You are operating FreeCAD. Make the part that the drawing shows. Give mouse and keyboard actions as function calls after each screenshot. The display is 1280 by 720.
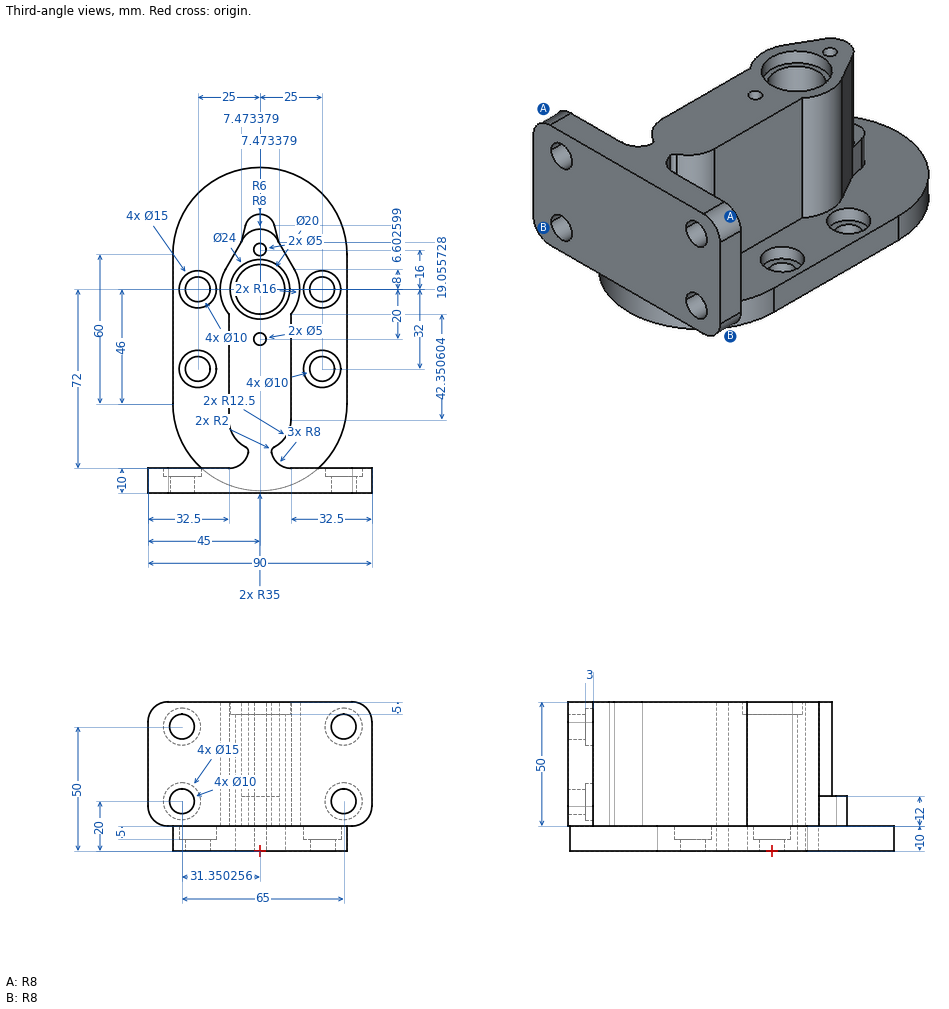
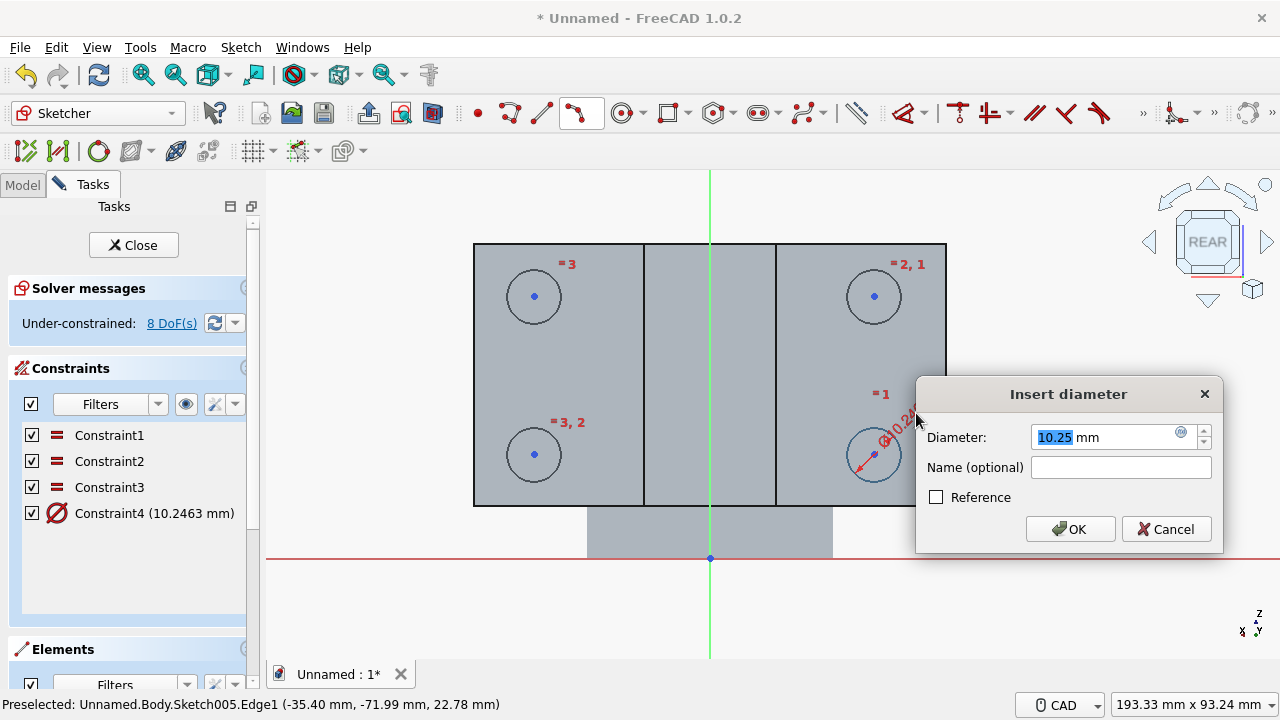
text(10)
key(Return)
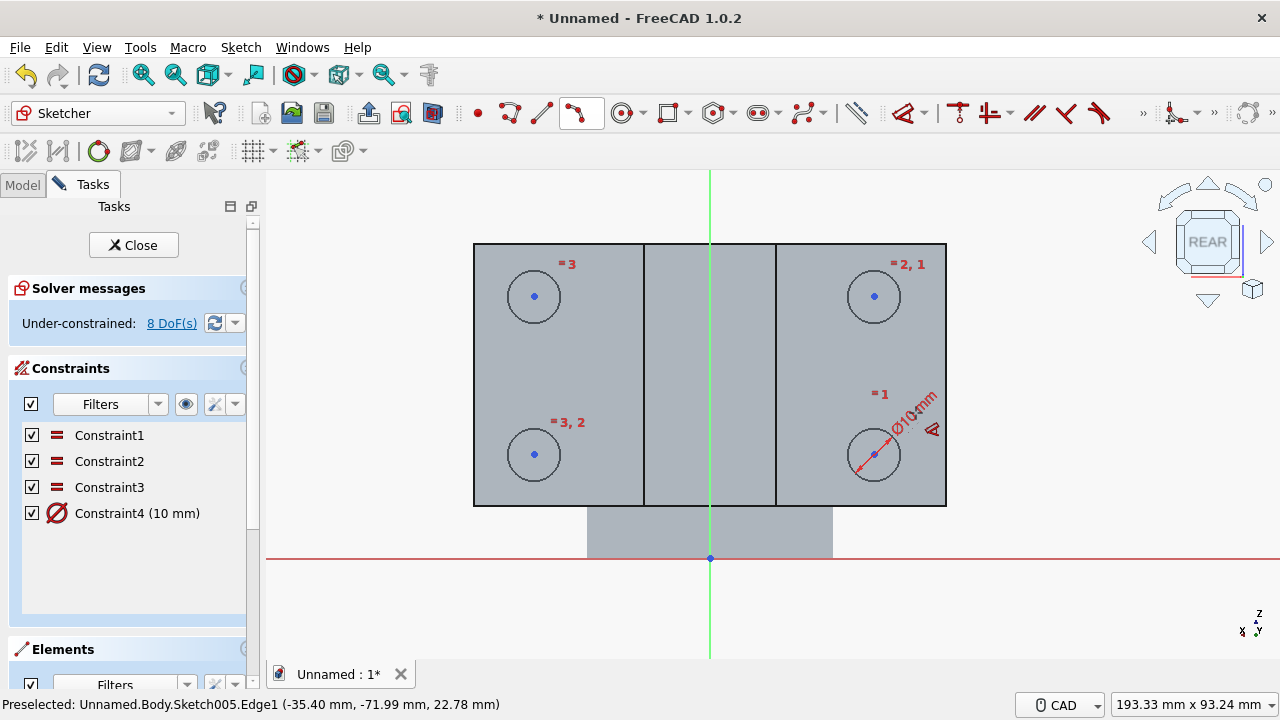
click(874, 455)
click(908, 507)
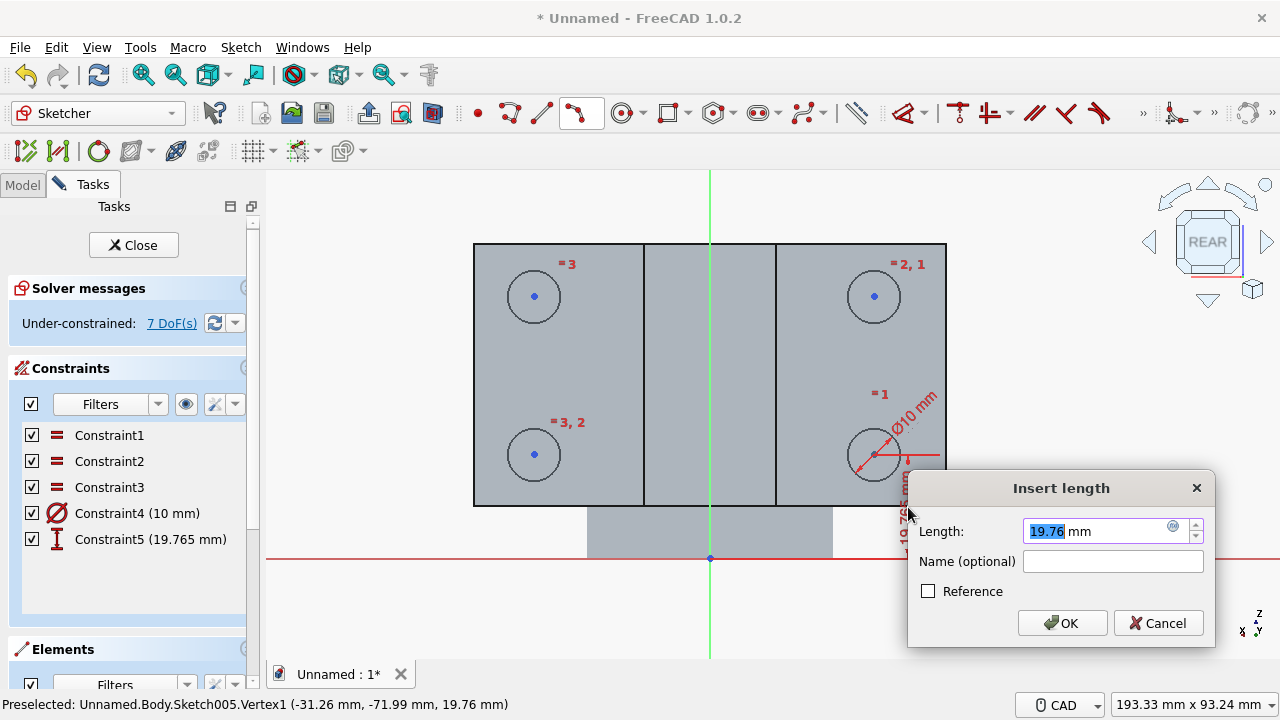
text(20)
key(Return)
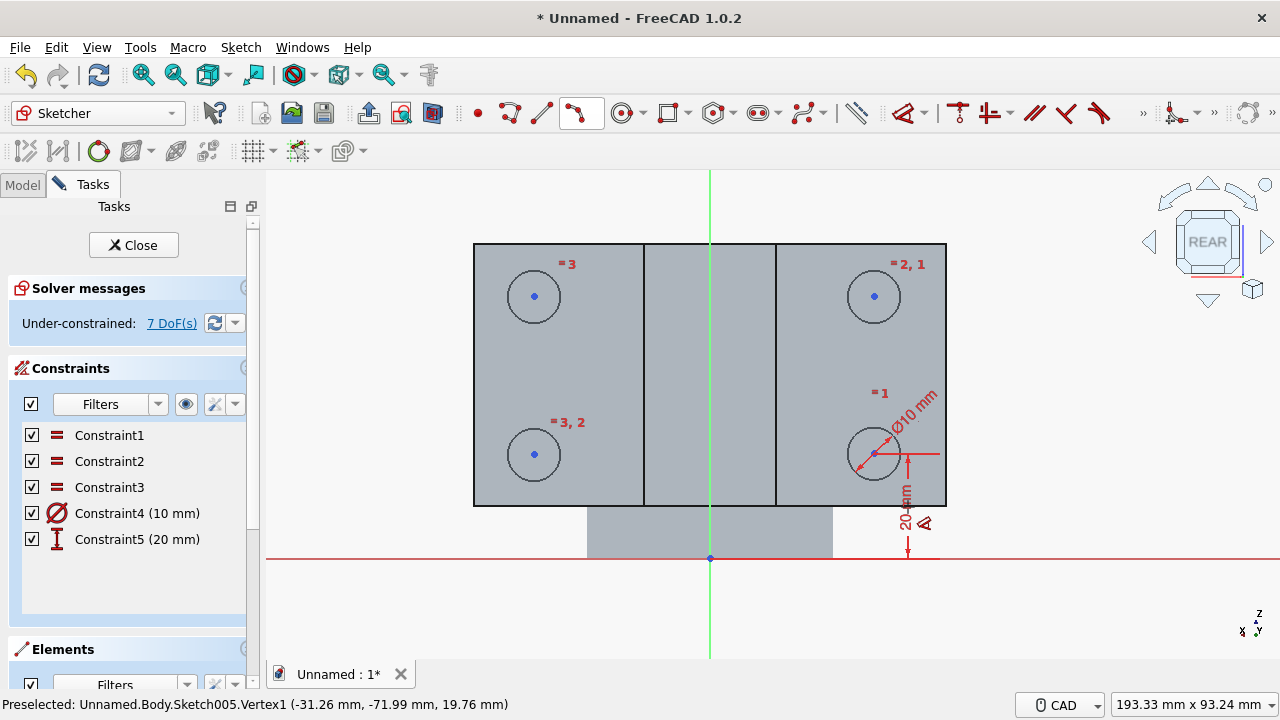
click(874, 297)
click(908, 368)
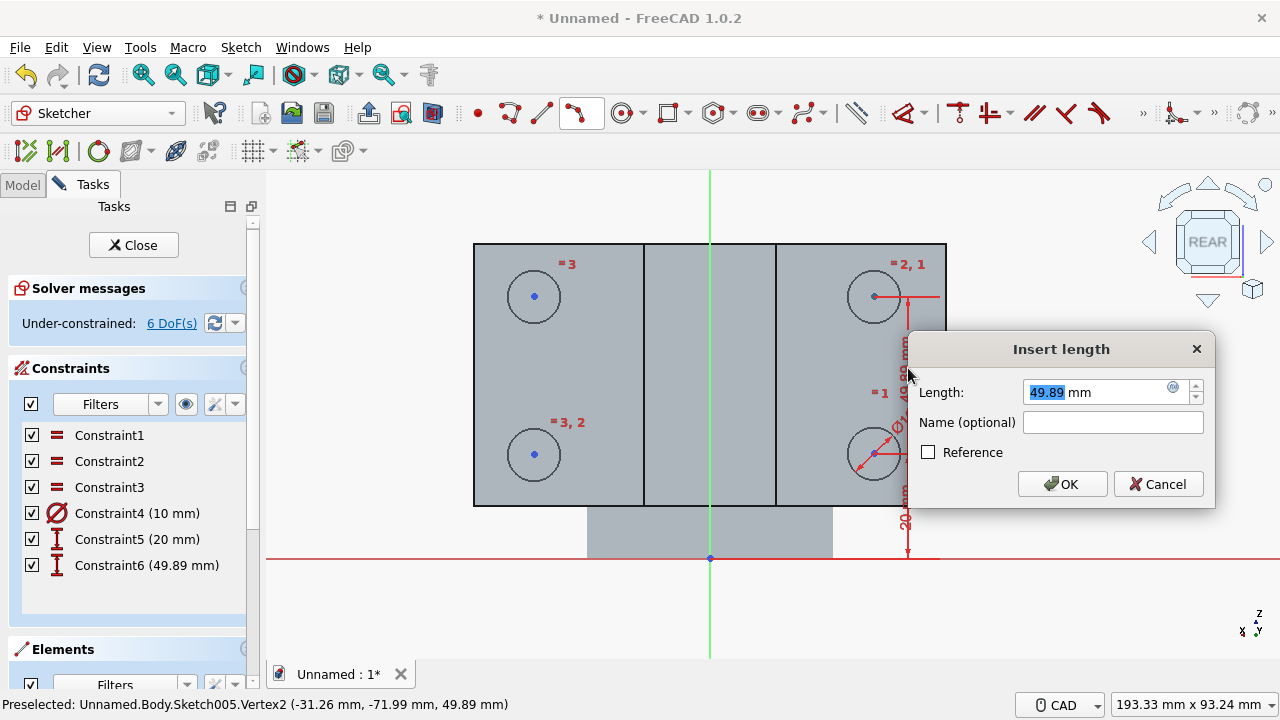
text(50)
key(Return)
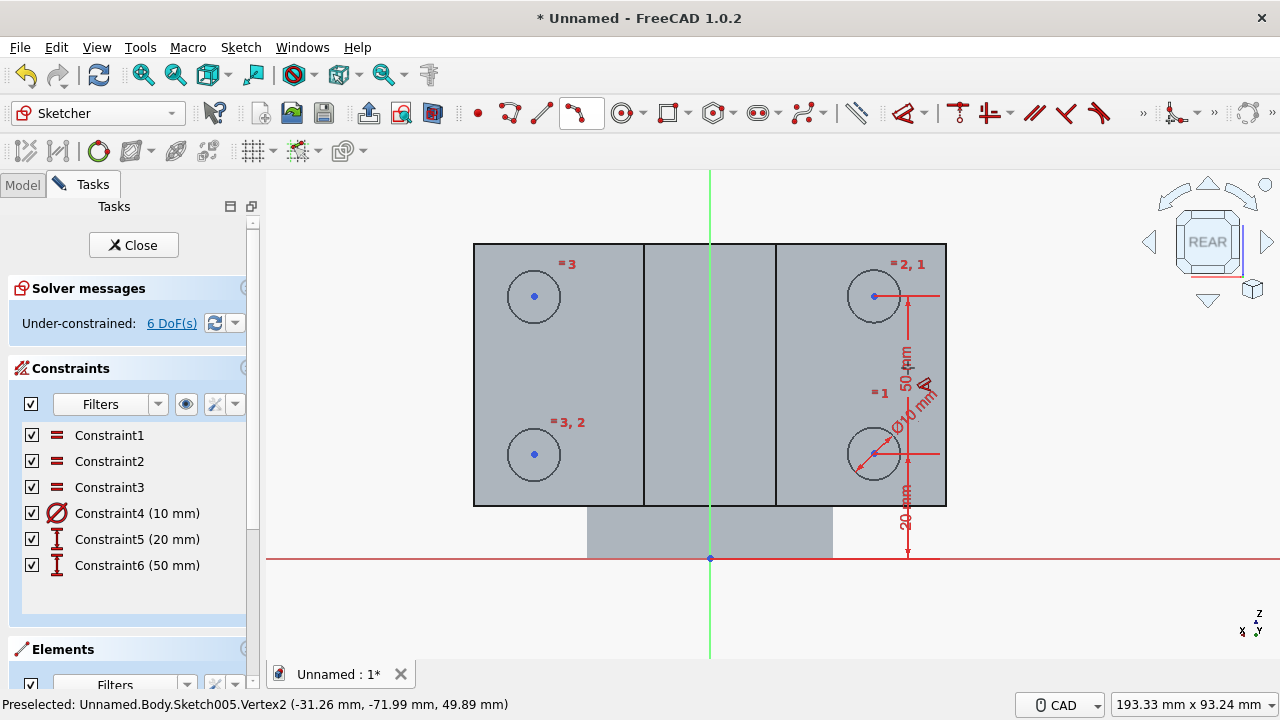
click(534, 455)
click(500, 507)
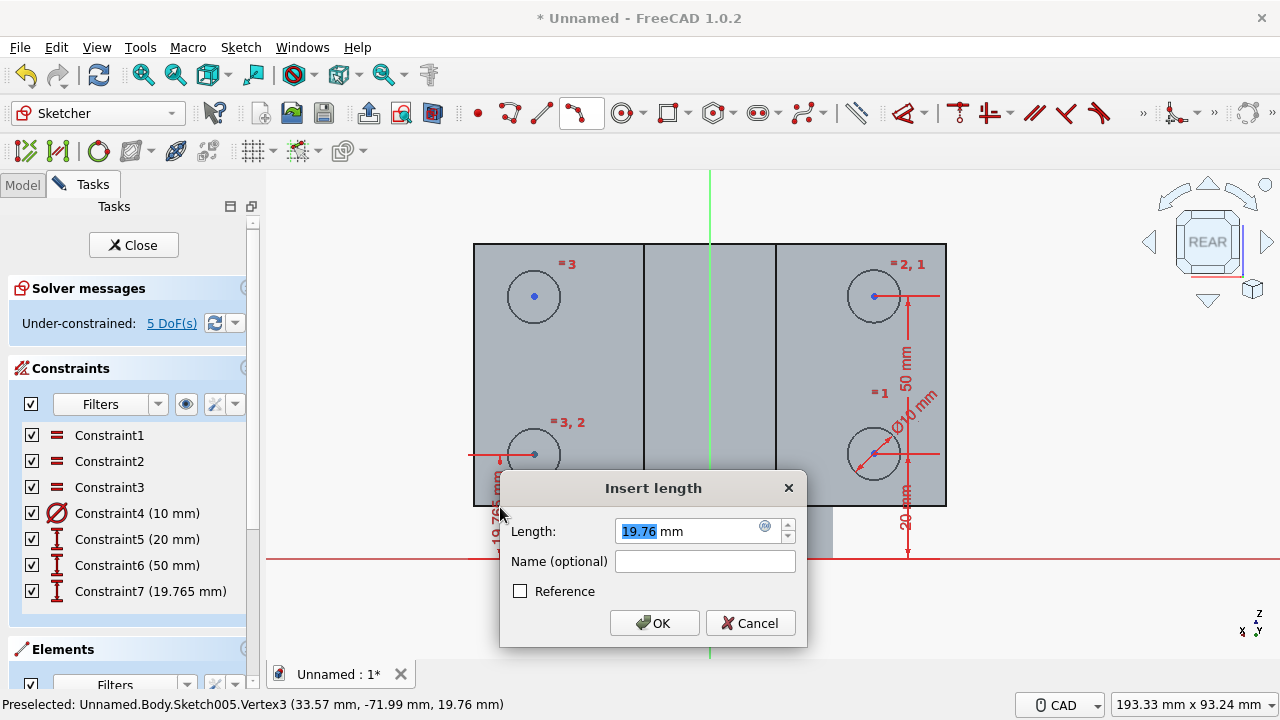
text(20)
key(Return)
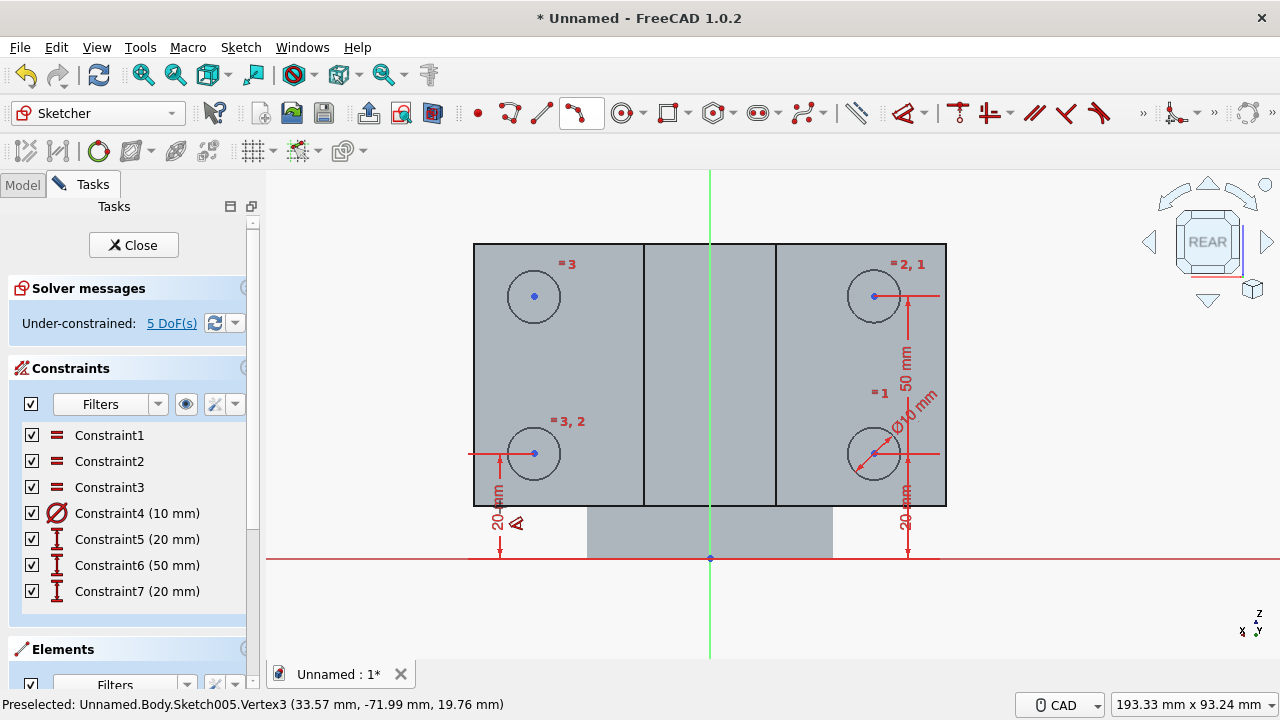
click(534, 297)
click(500, 428)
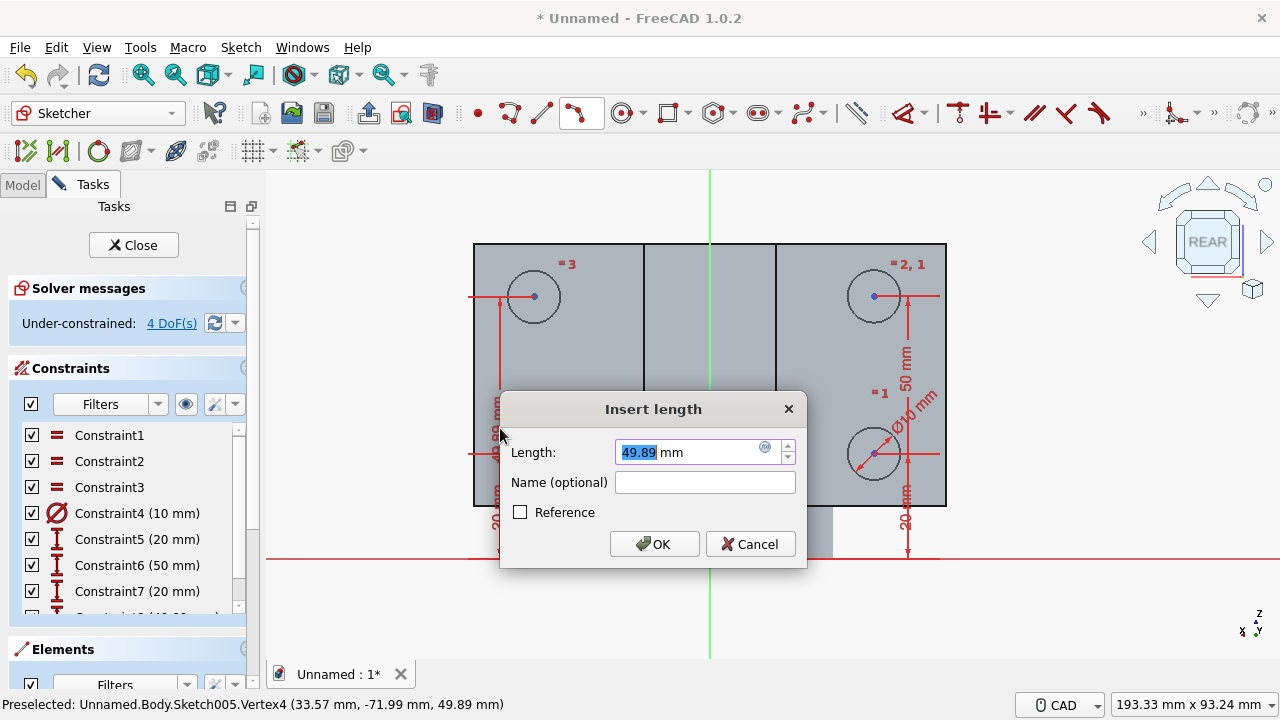
text(50)
key(Return)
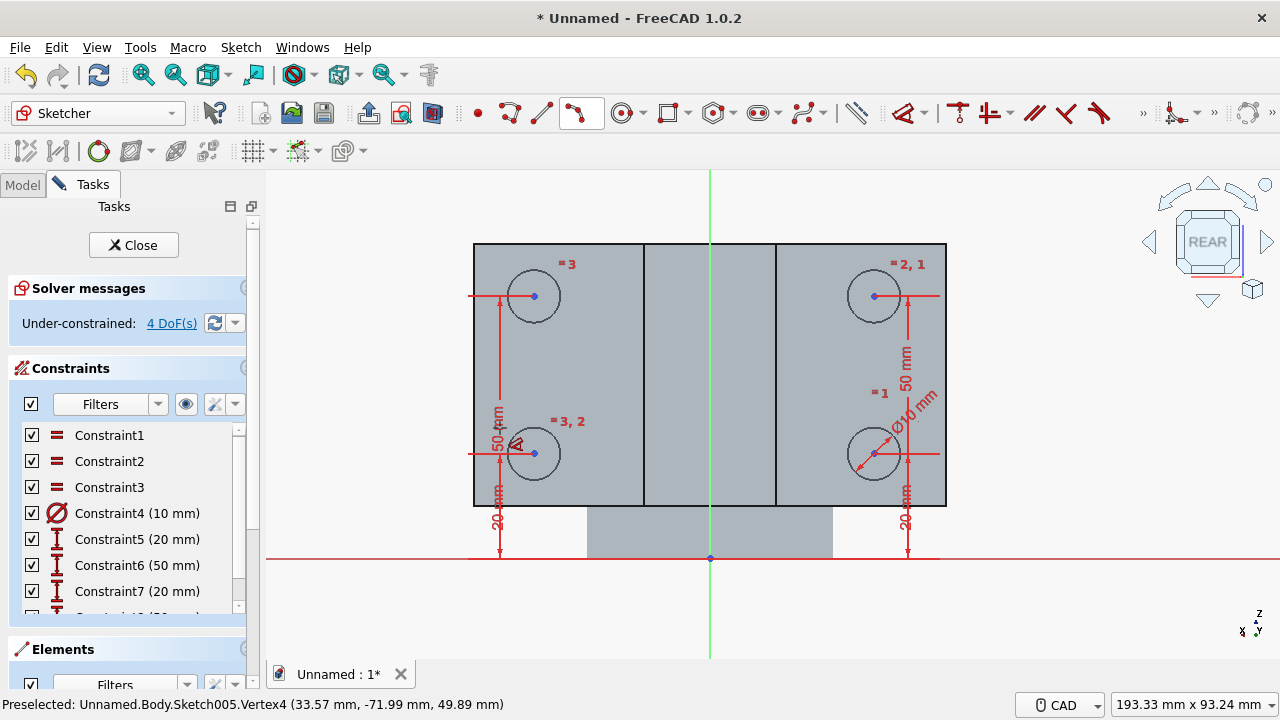
click(874, 454)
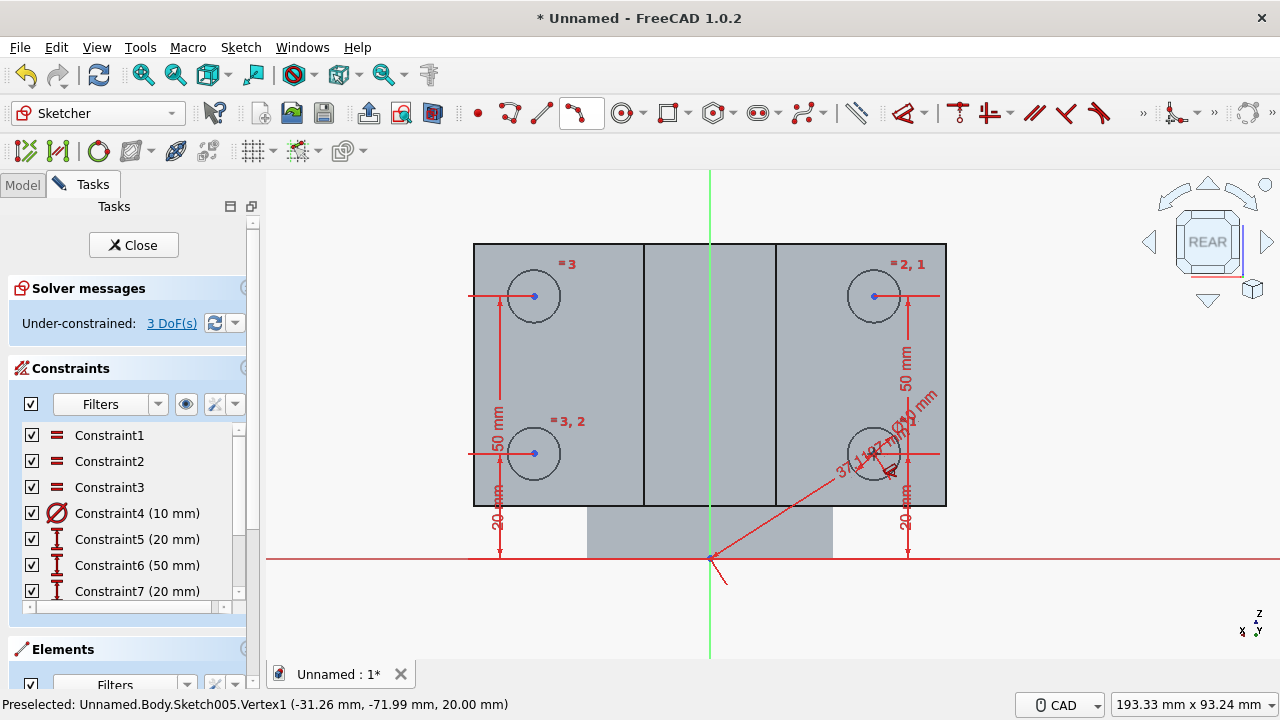
click(534, 454)
click(626, 488)